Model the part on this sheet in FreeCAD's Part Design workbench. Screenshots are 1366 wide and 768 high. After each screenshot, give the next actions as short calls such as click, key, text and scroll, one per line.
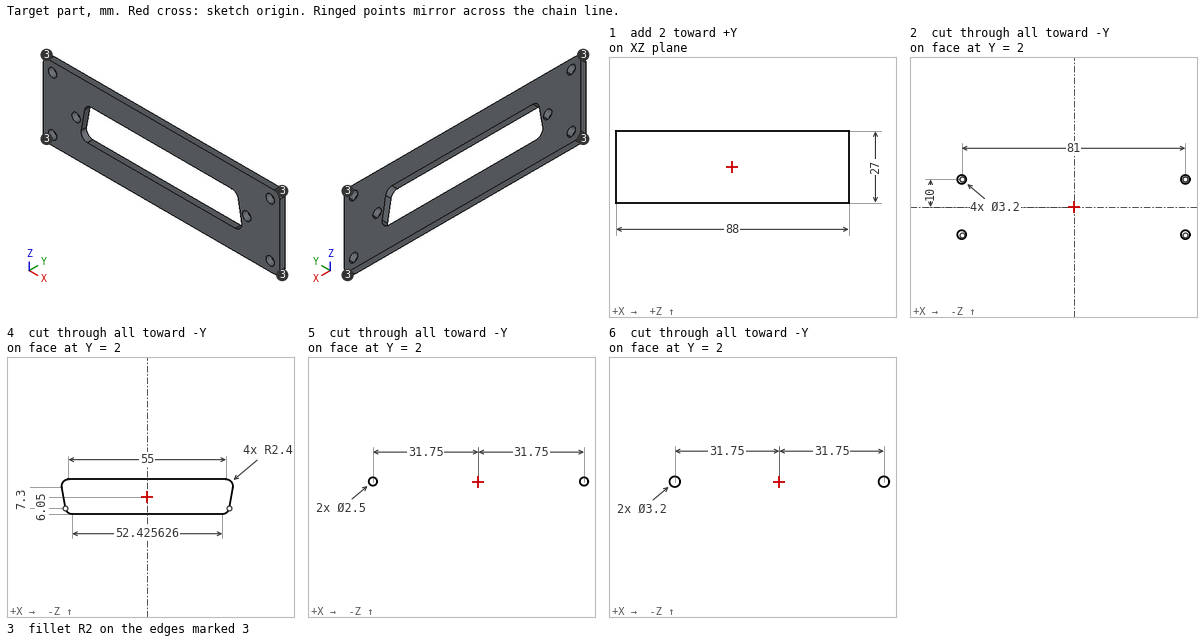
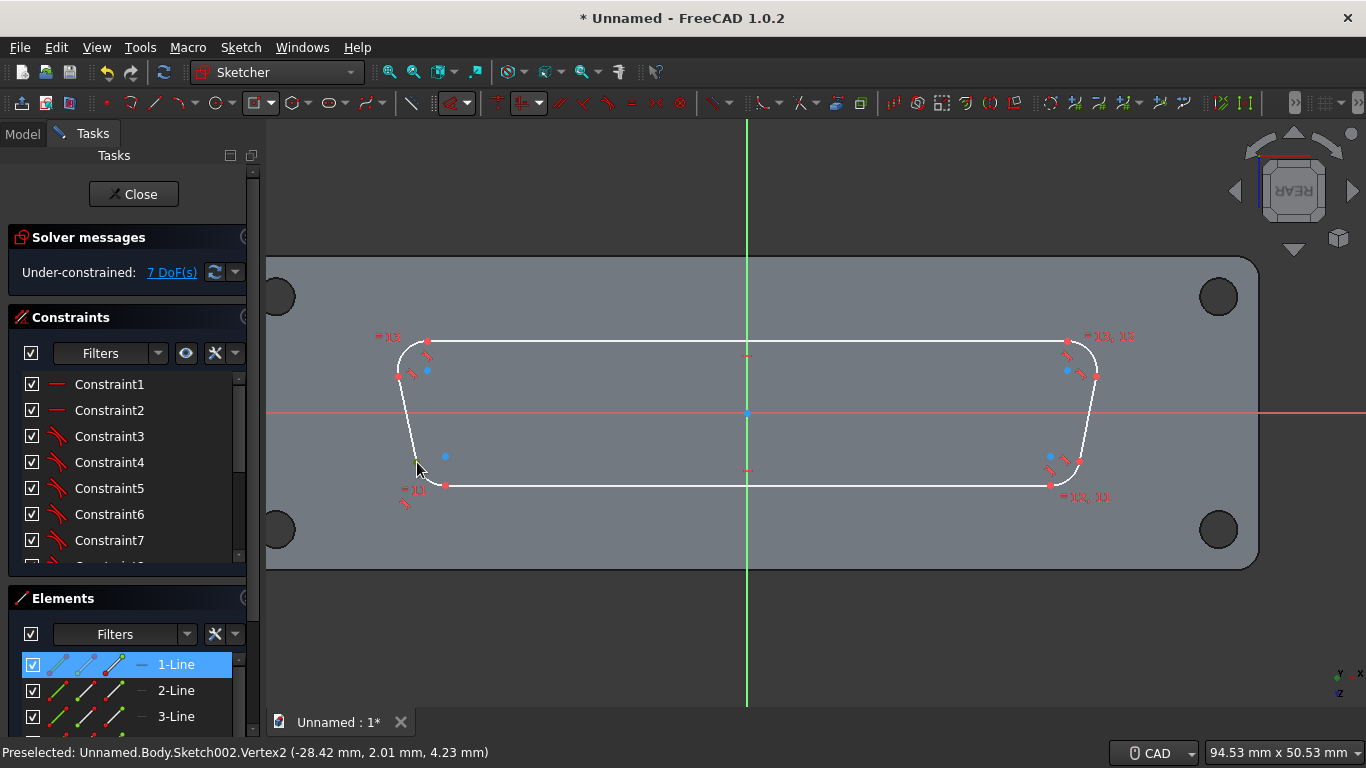
click(1080, 462)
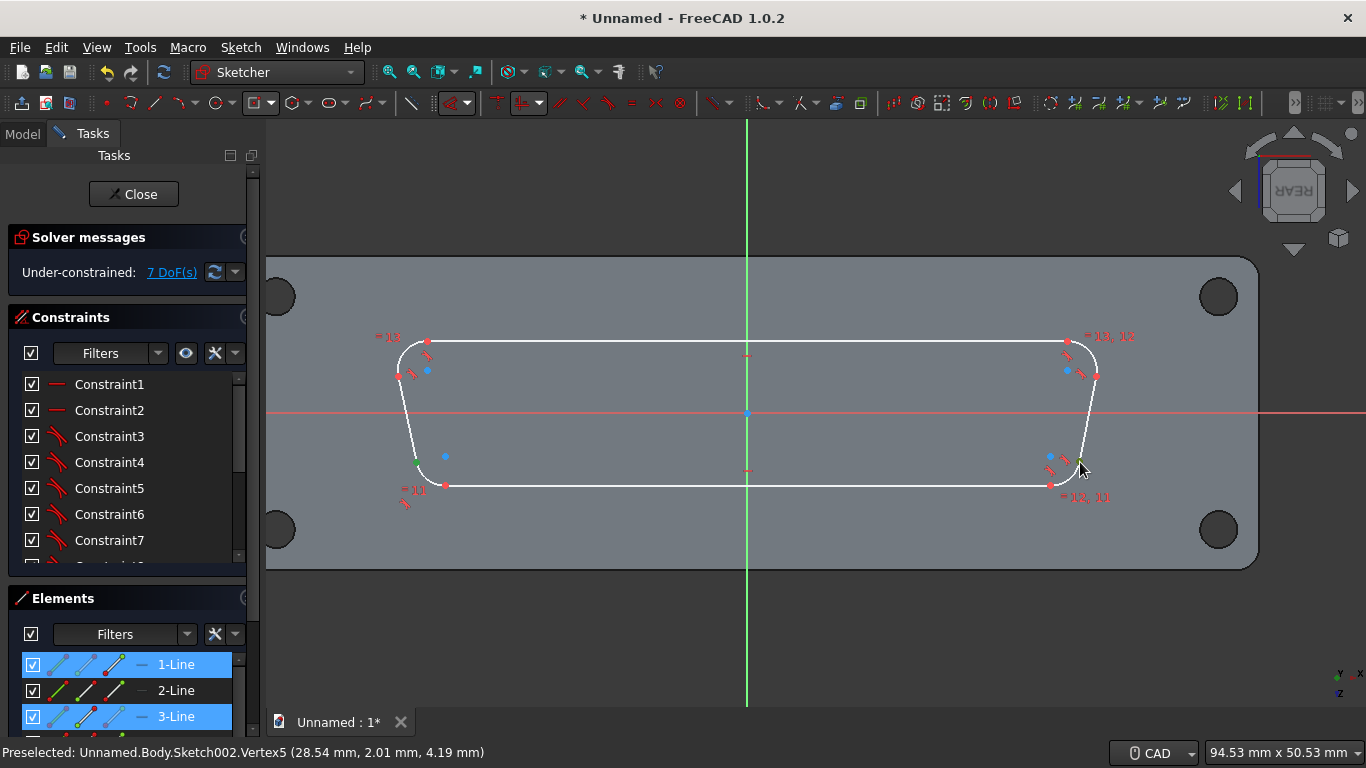
click(747, 641)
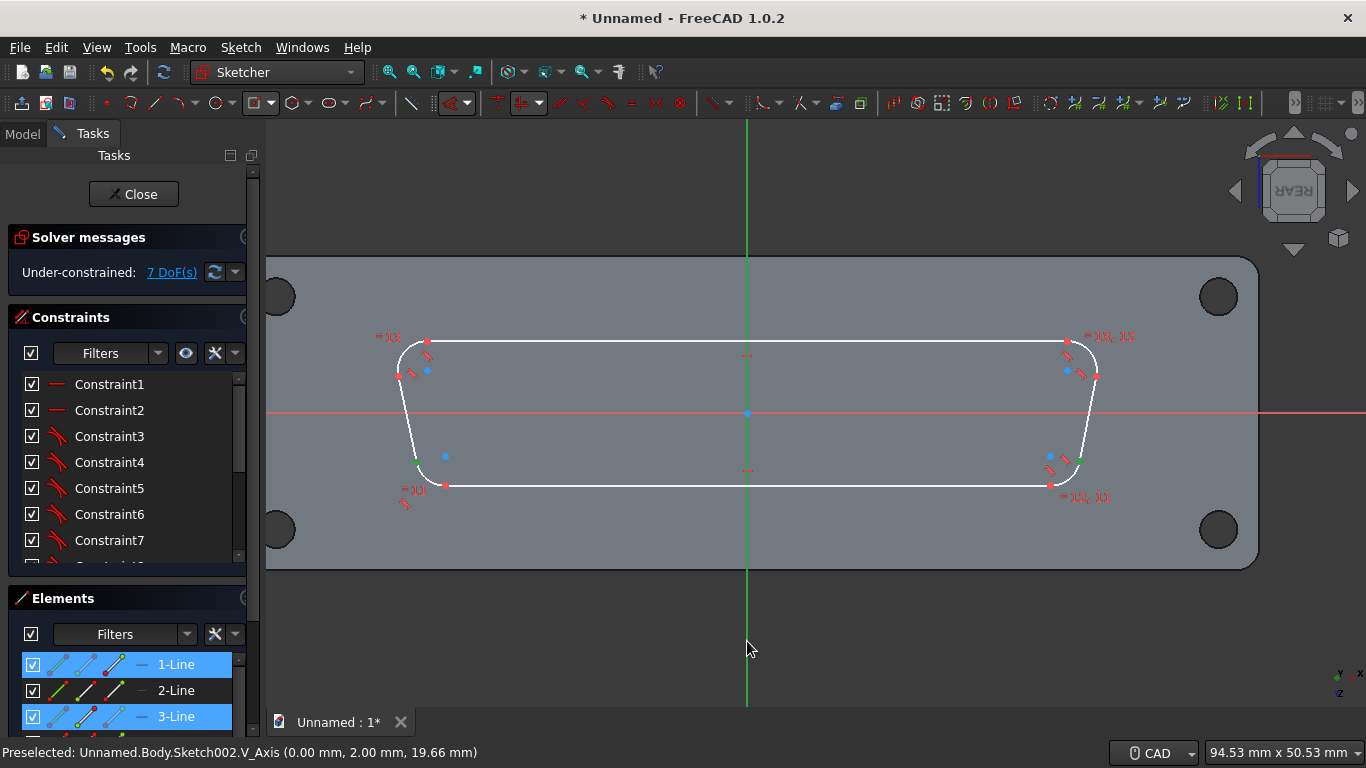
key(s)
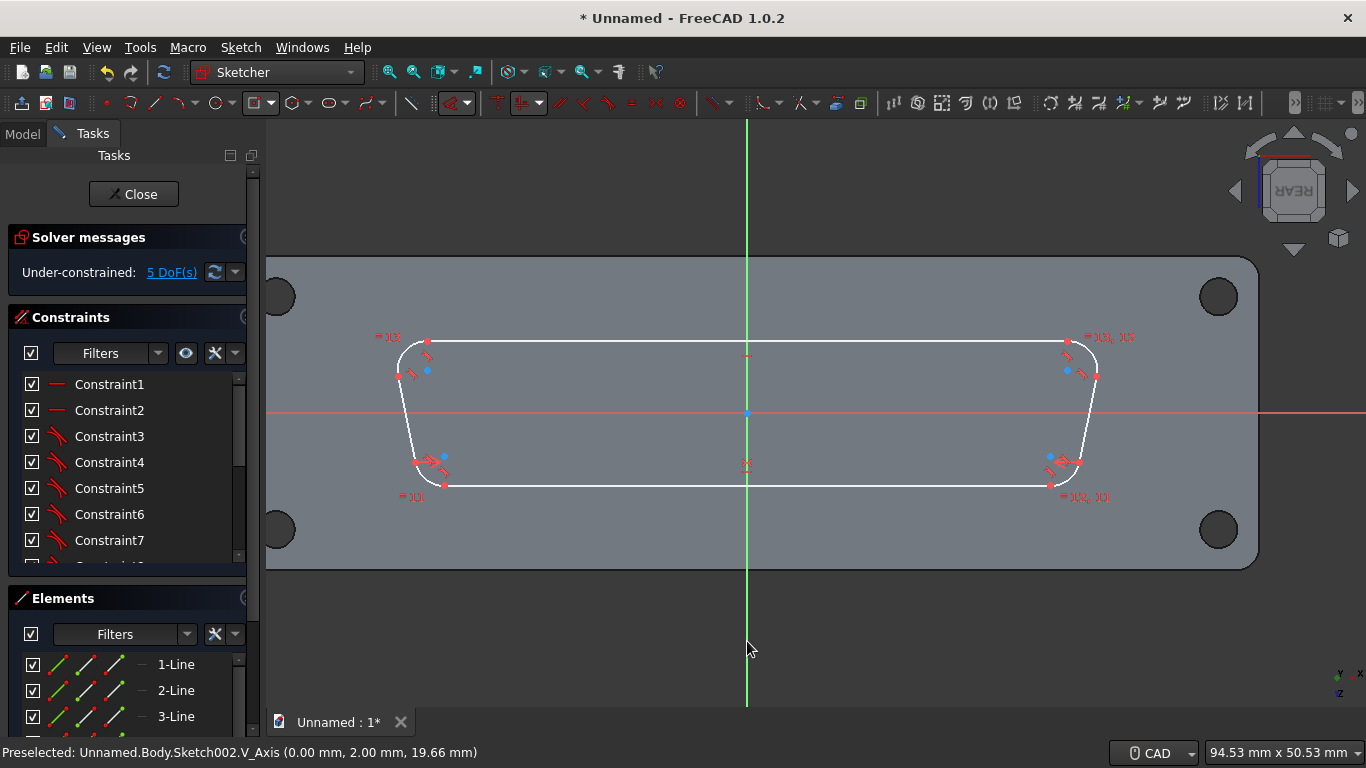
scroll(420, 473, up, 2)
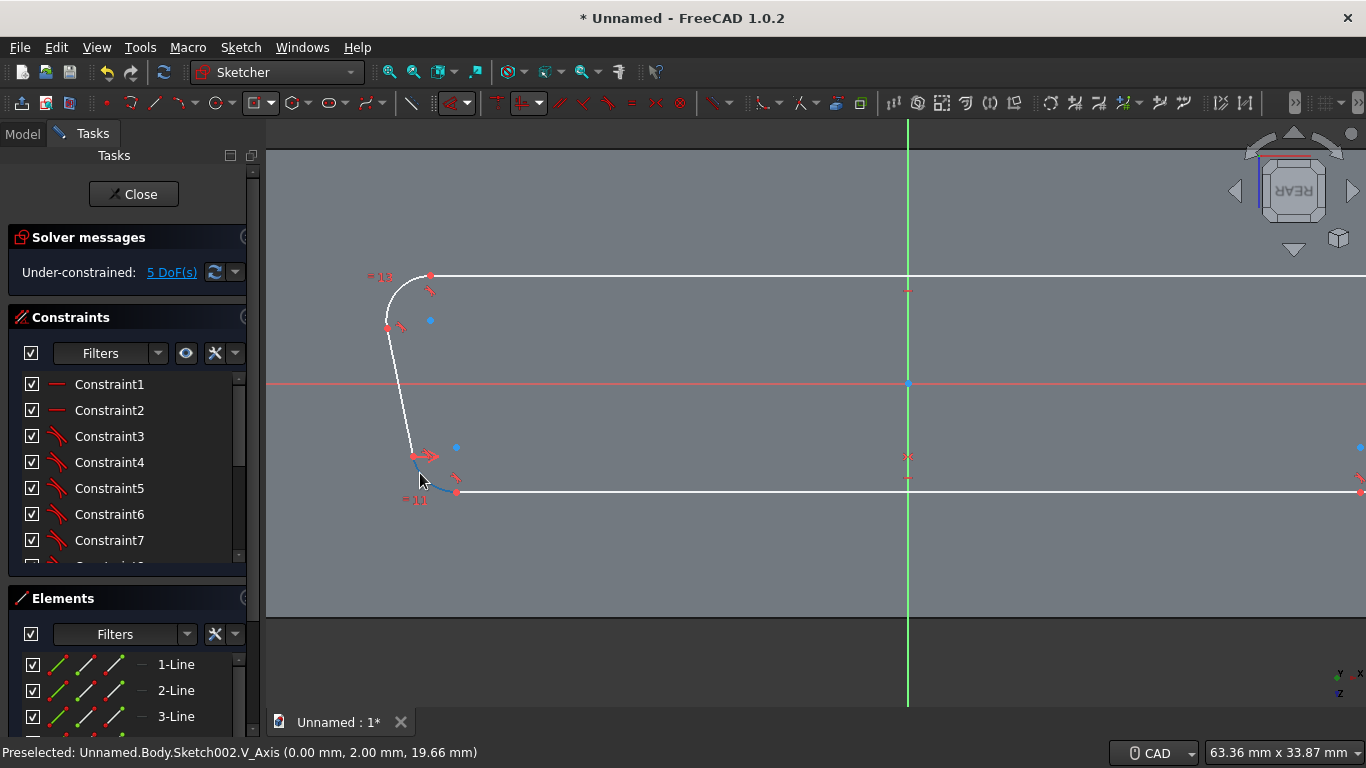
click(420, 473)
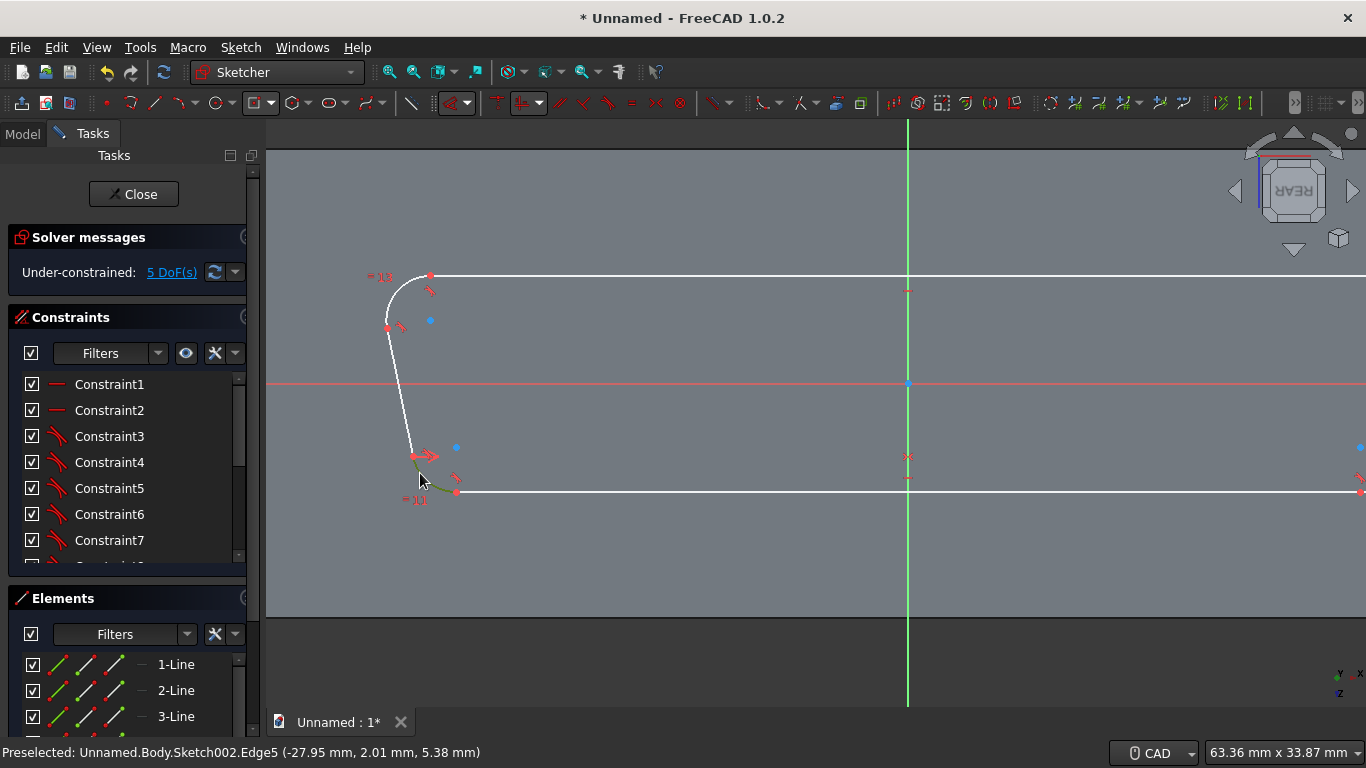
key(k)
key(r)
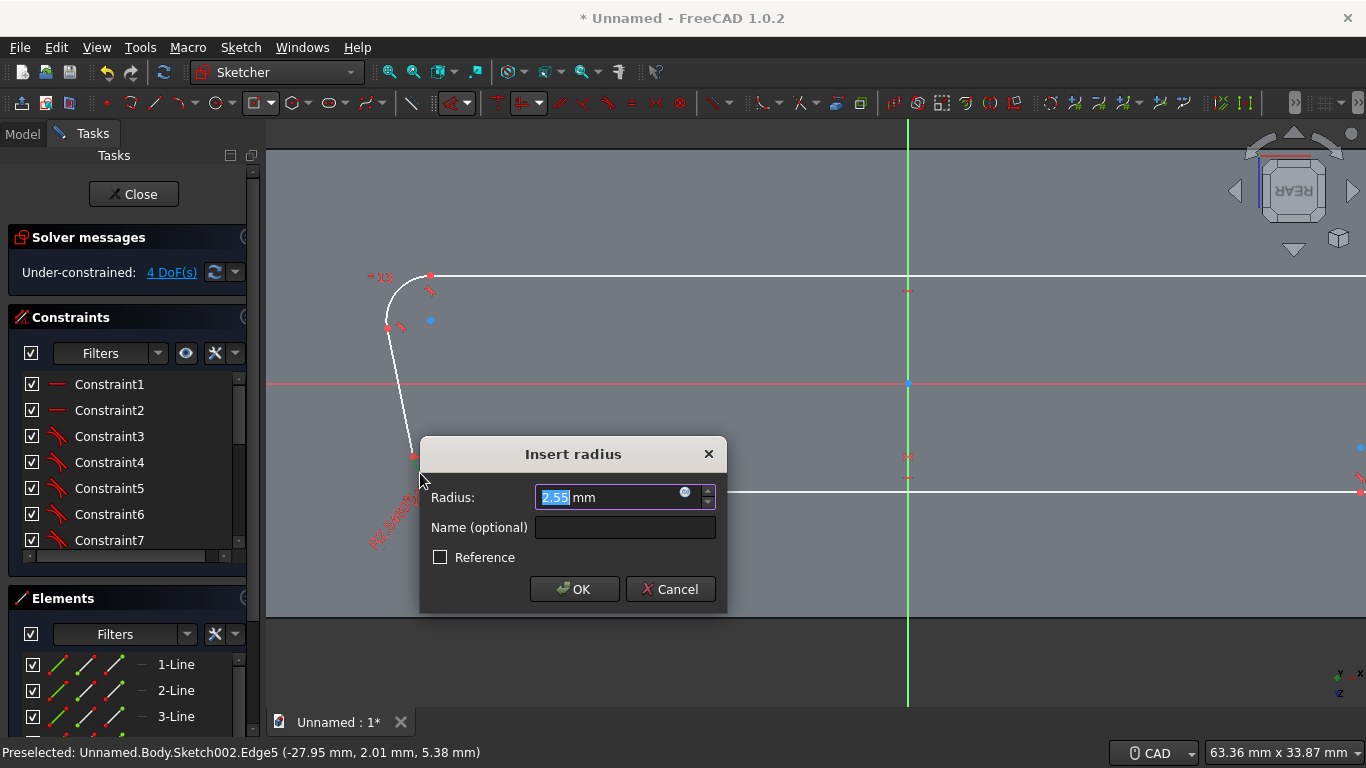
text(2.4)
key(Return)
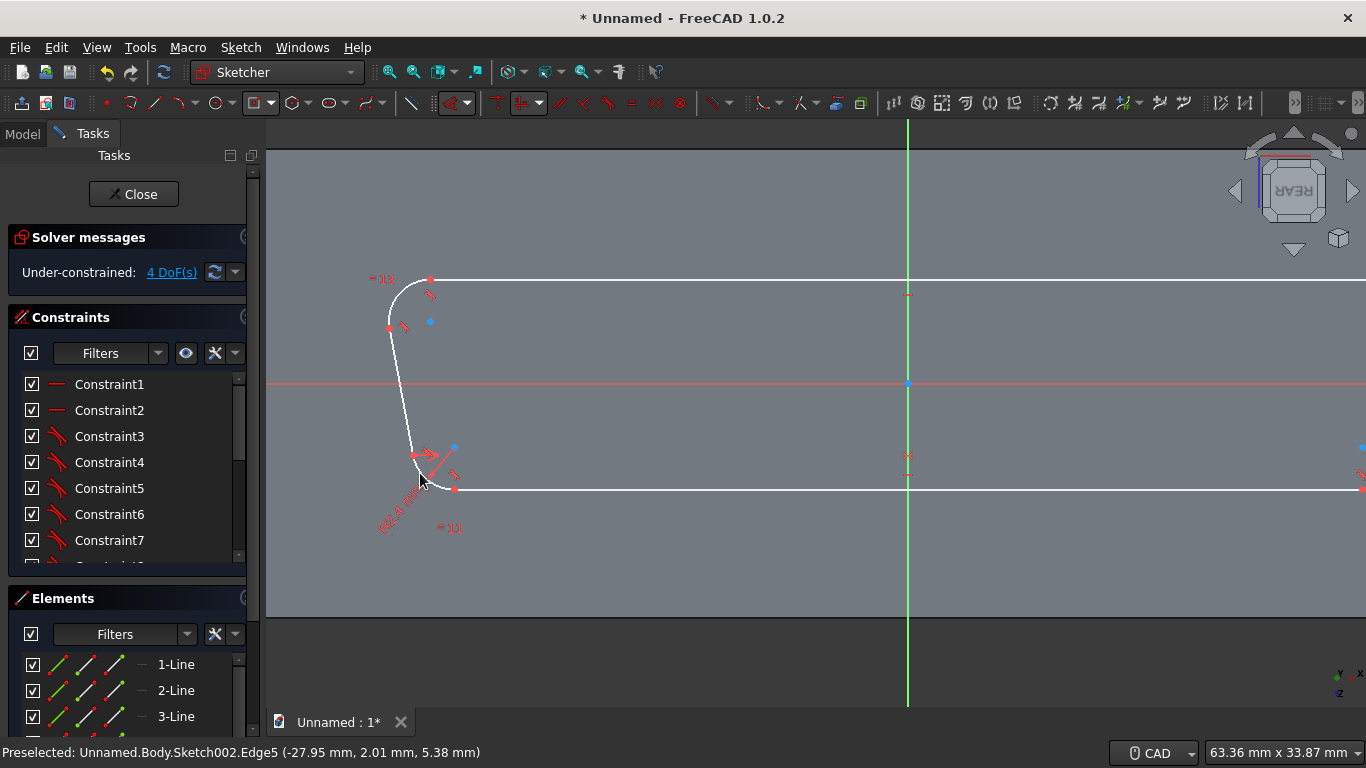
click(1100, 280)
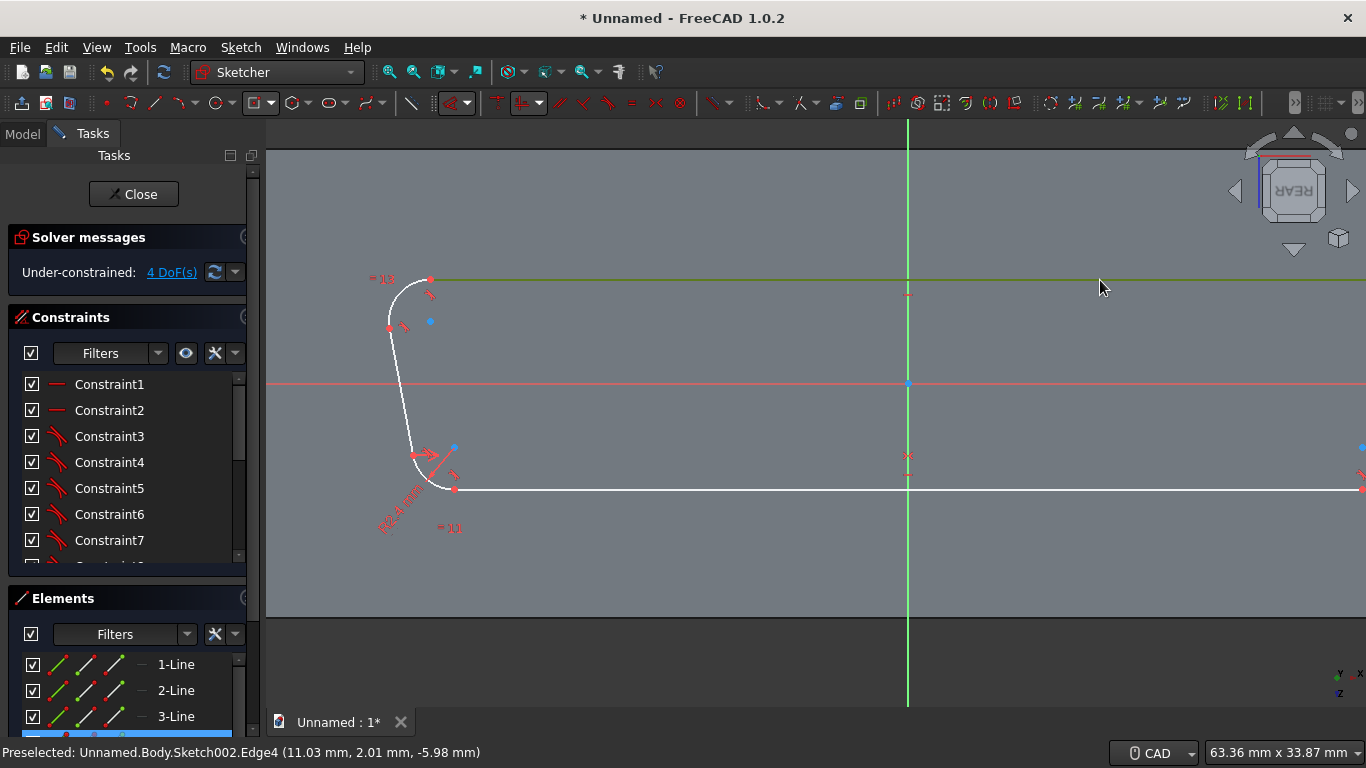
key(l)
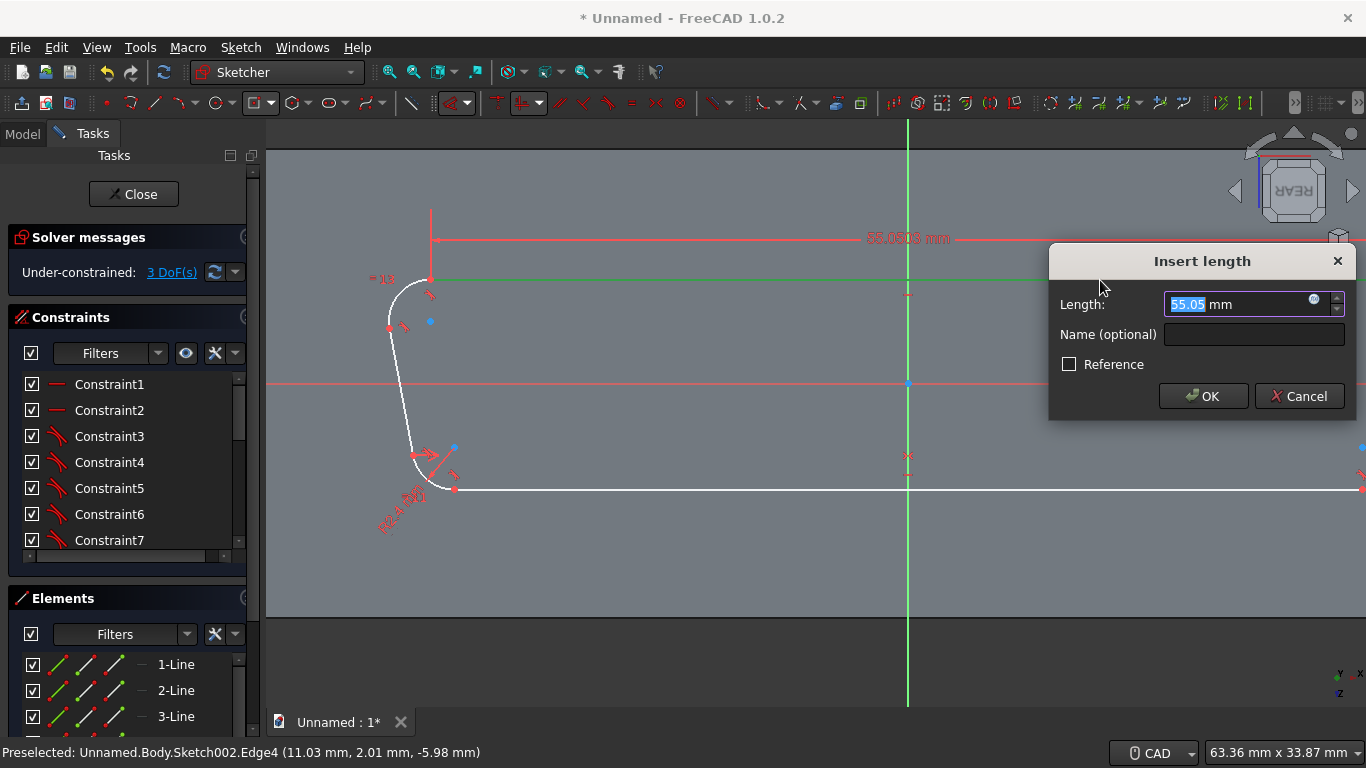
text(55)
key(Return)